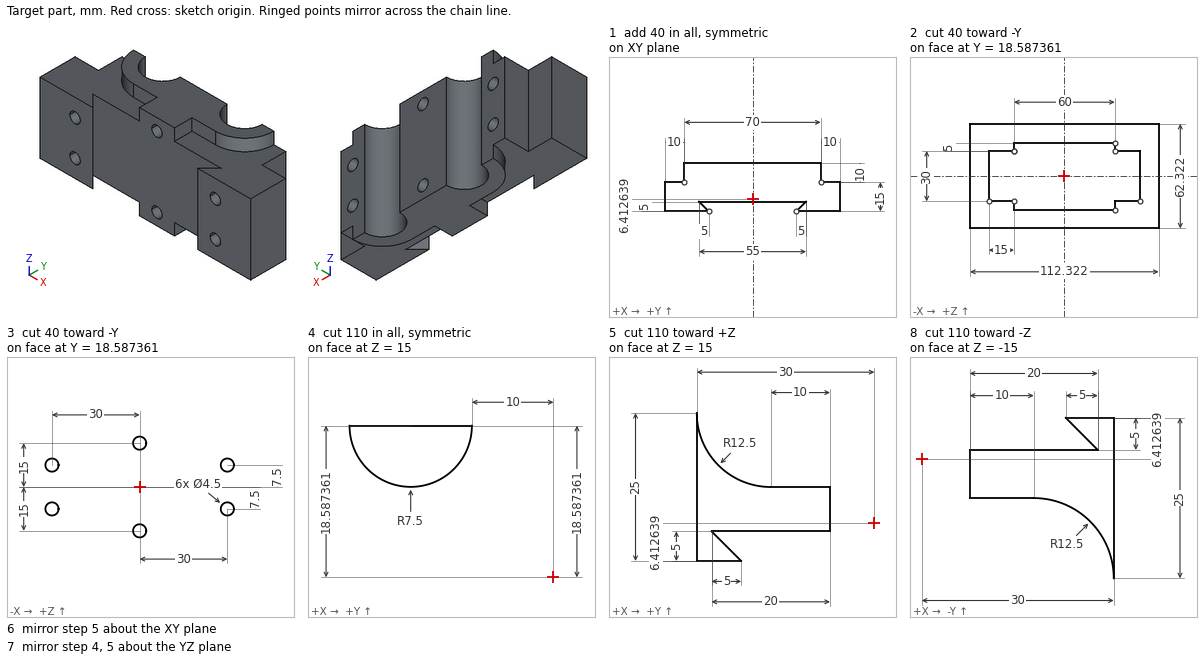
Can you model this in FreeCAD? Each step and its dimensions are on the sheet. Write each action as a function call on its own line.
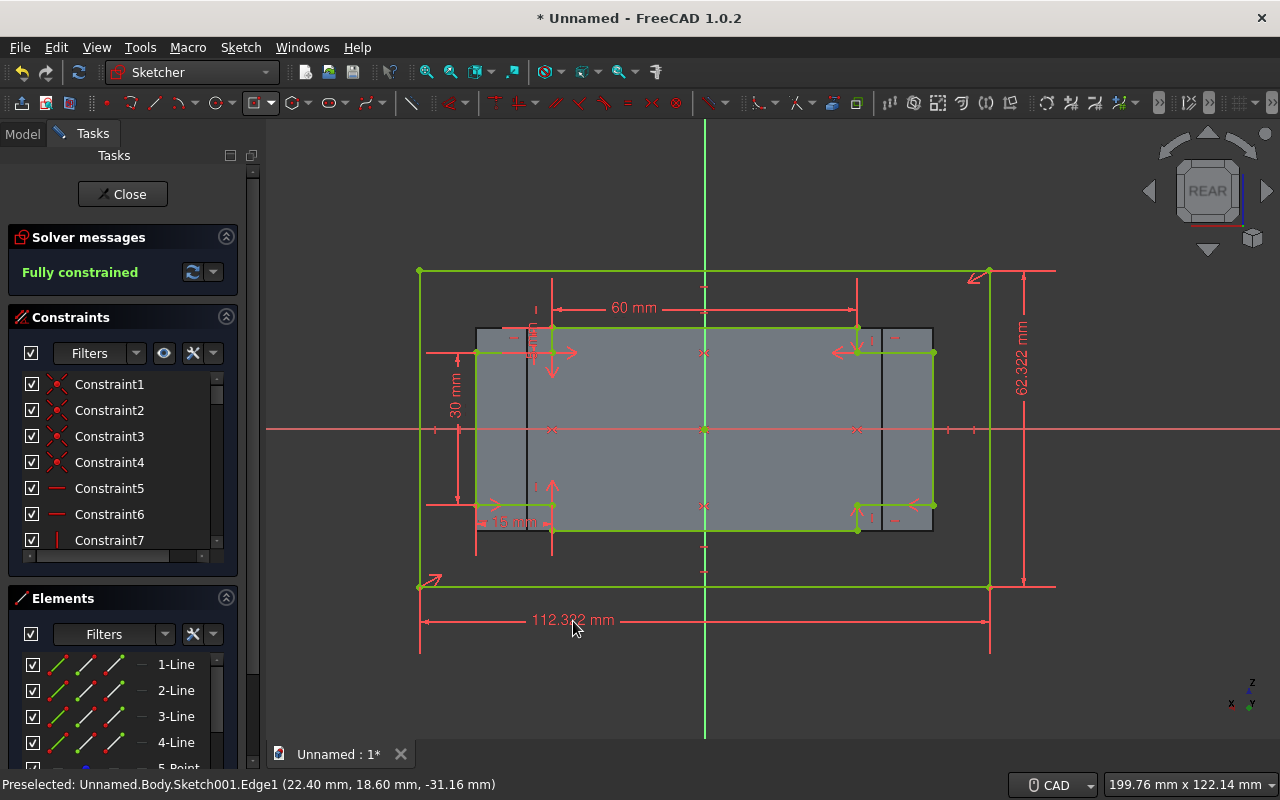
click(123, 194)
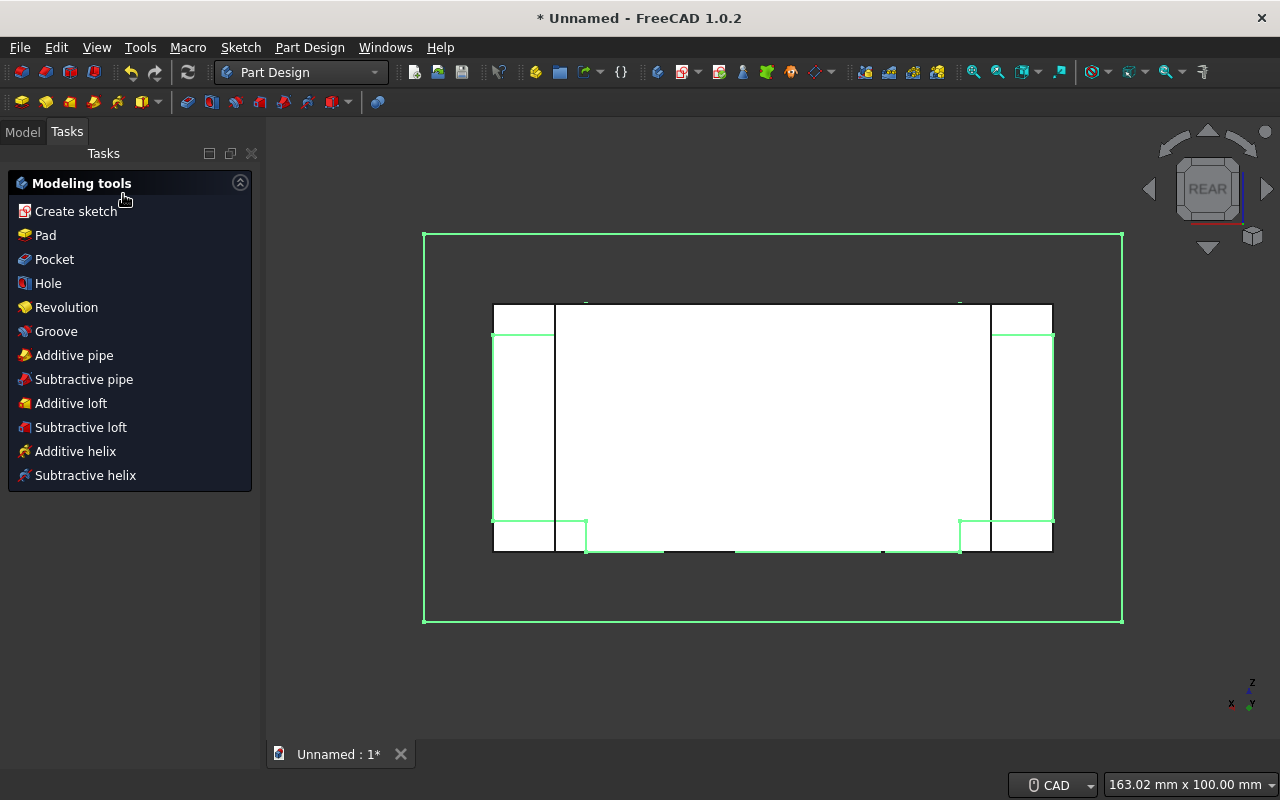
click(188, 102)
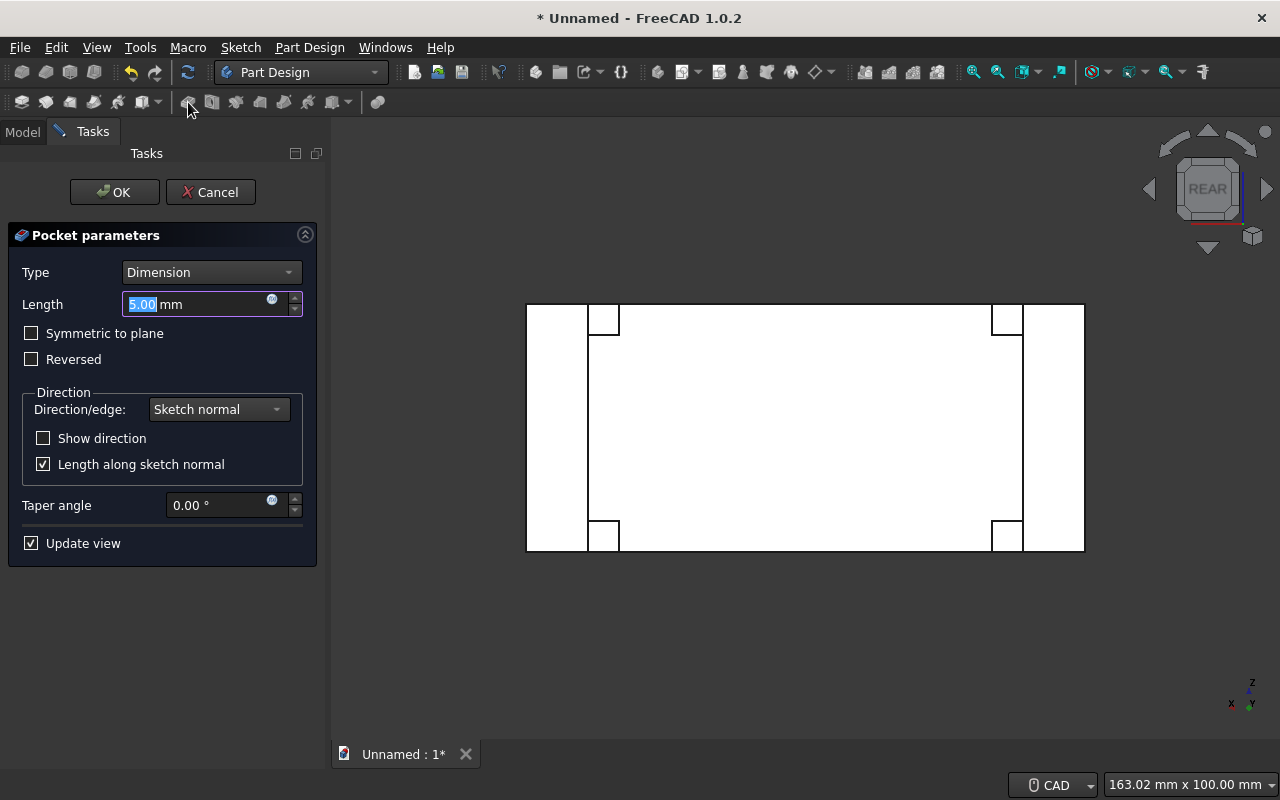
text(40)
key(Tab)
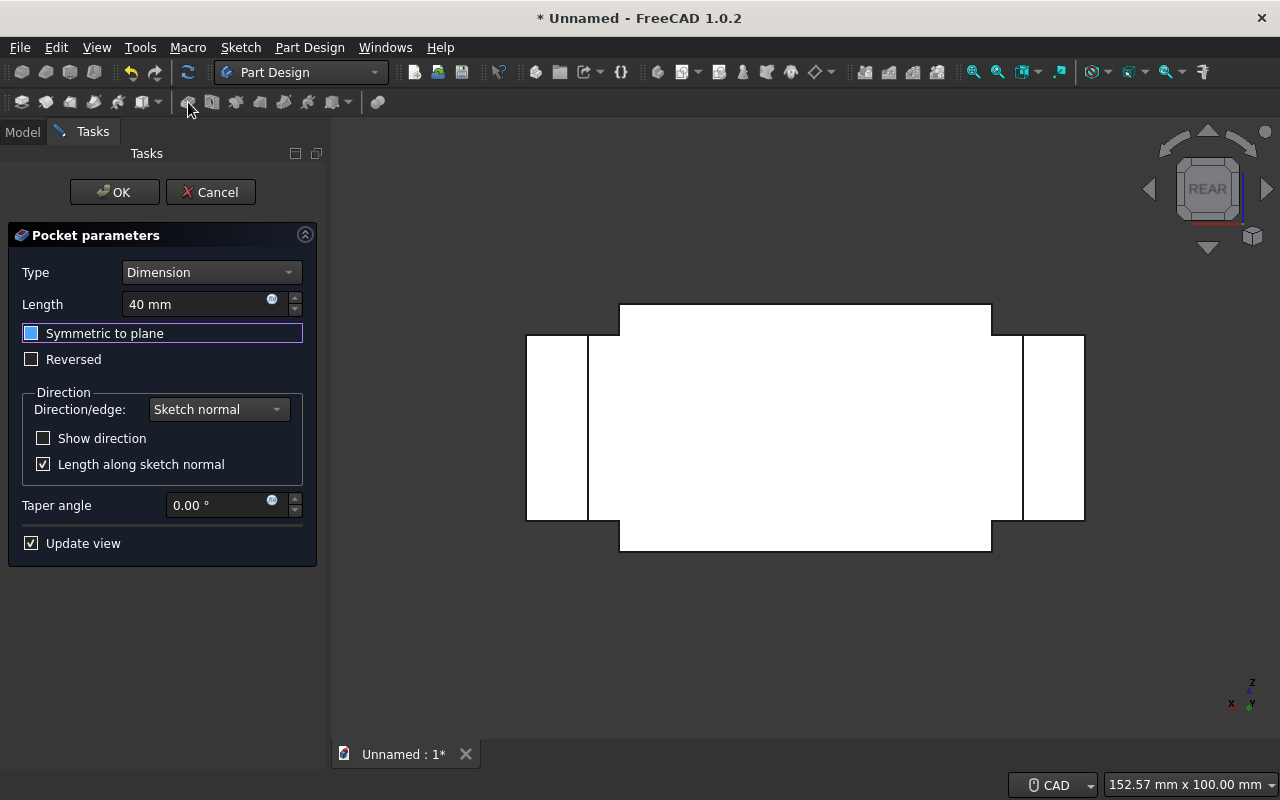
click(115, 192)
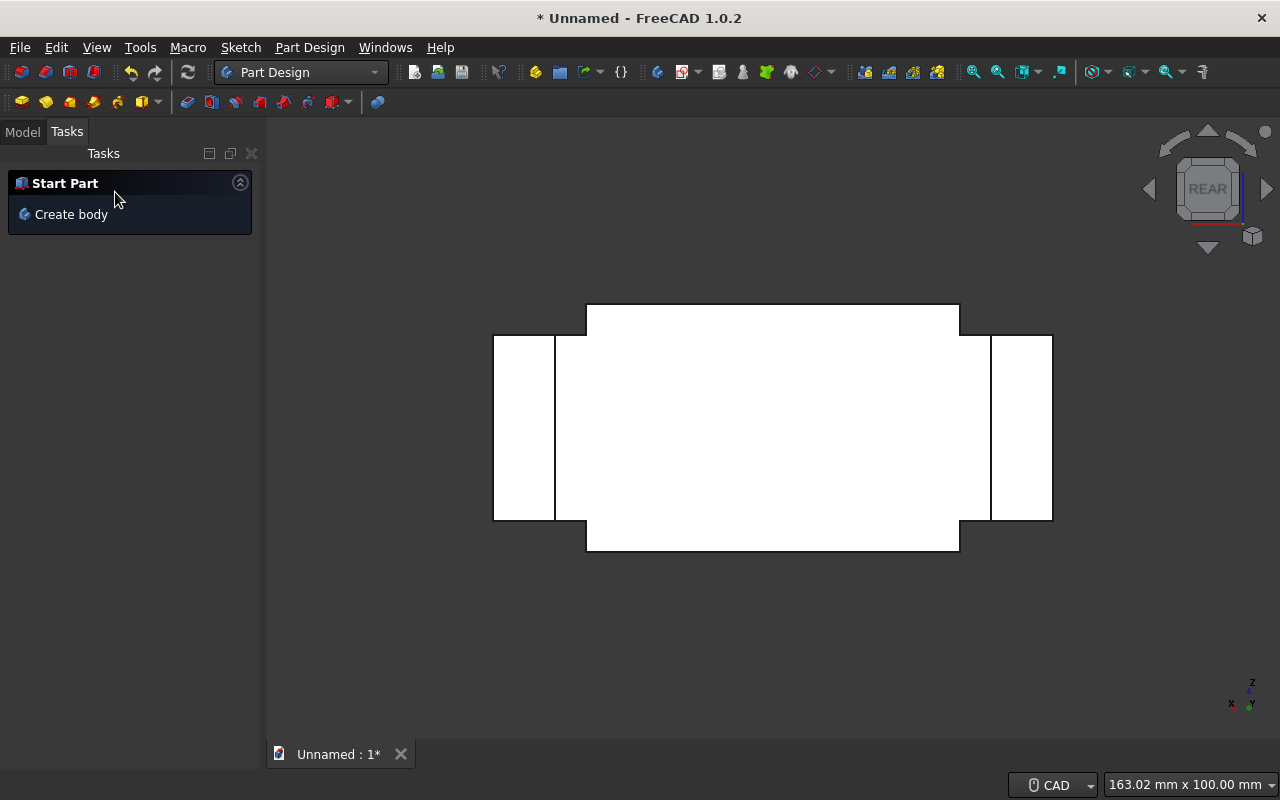
click(711, 427)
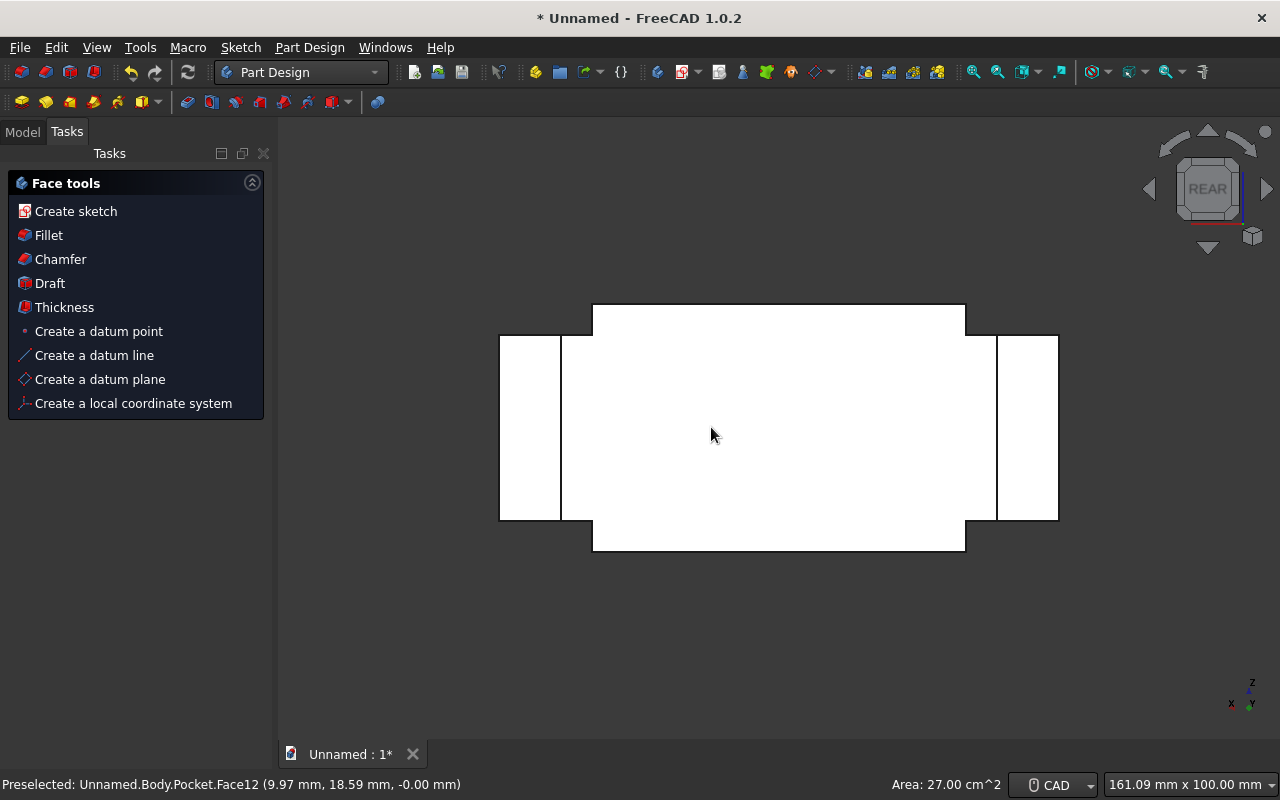
click(682, 72)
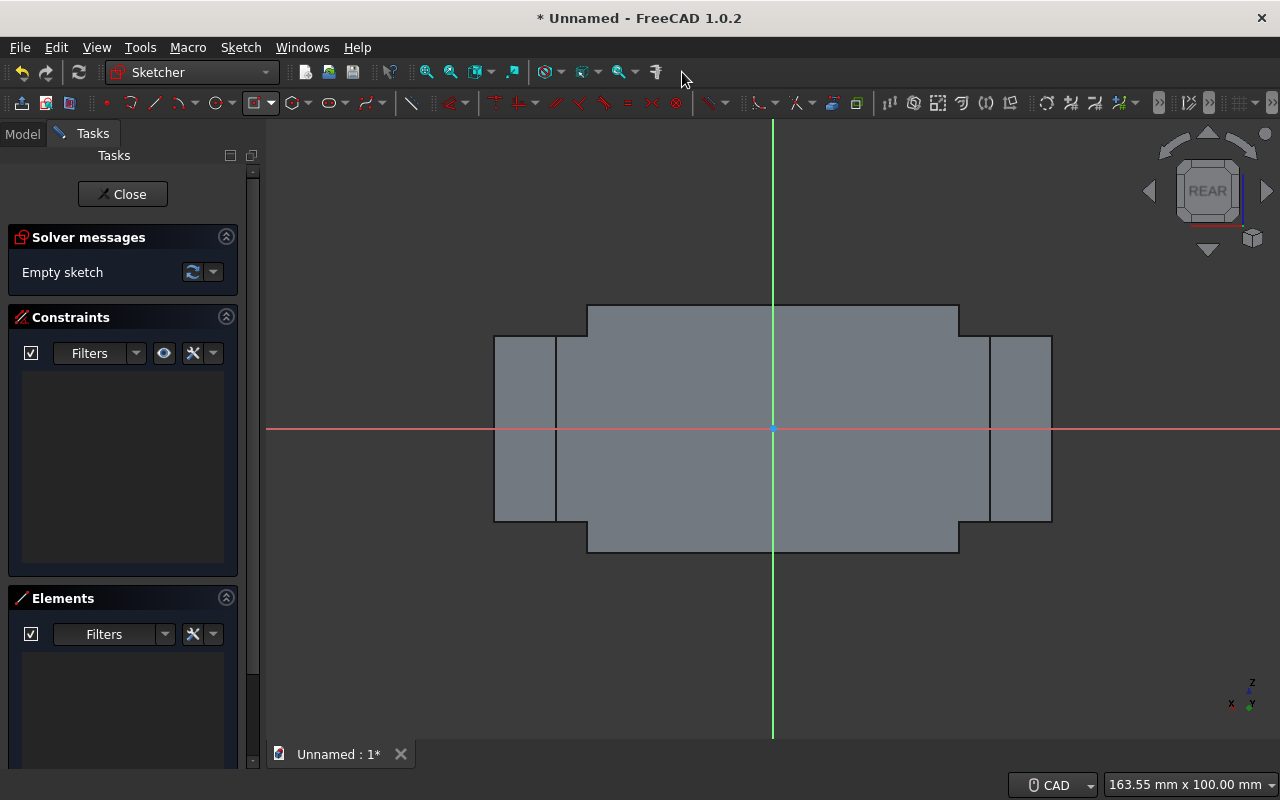
scroll(912, 429, up, 2)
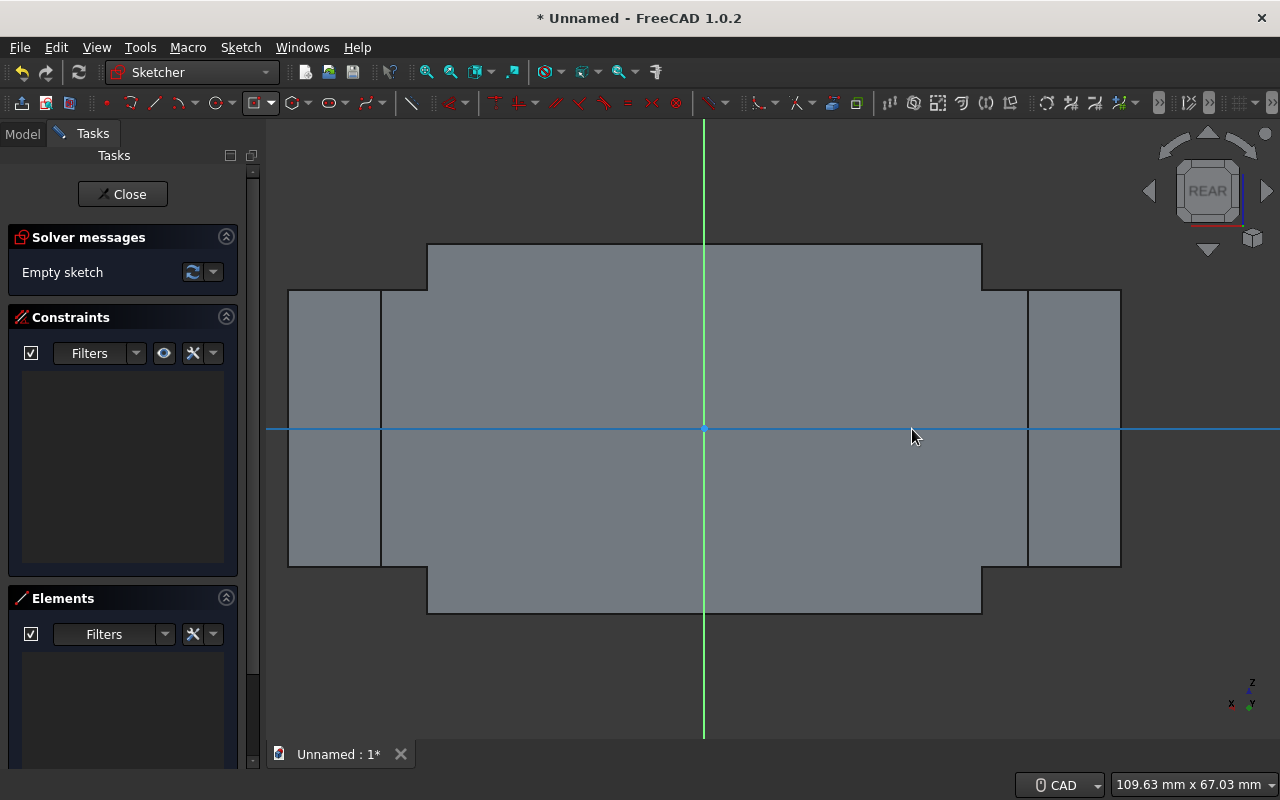
key(g)
key(c)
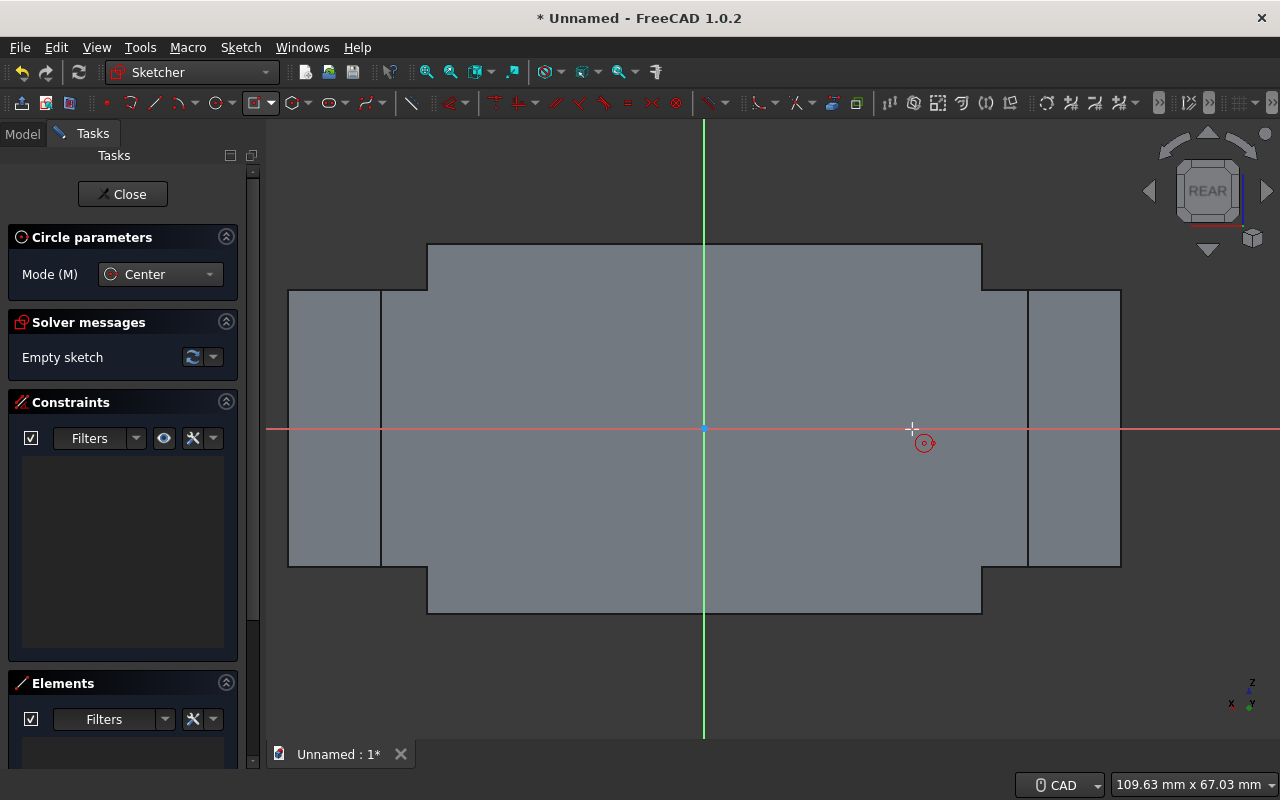
click(982, 498)
click(997, 483)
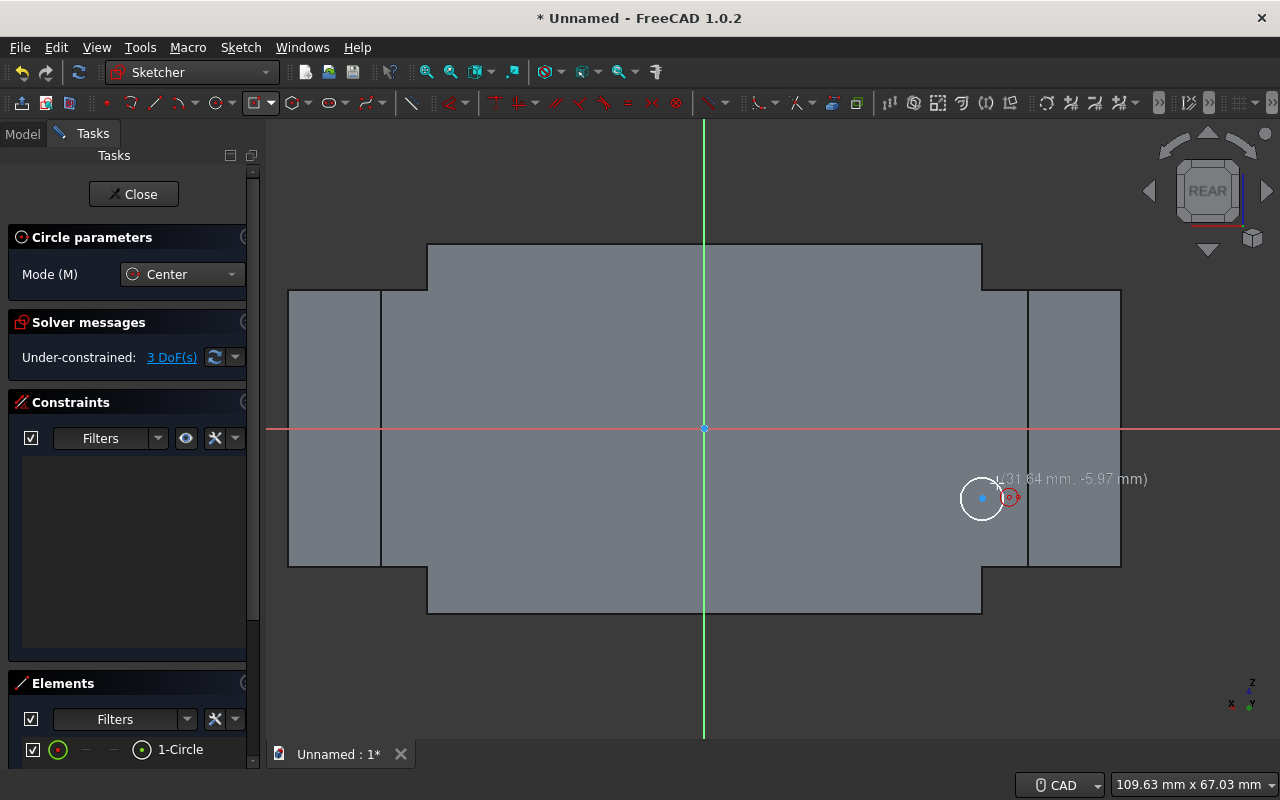
click(982, 359)
click(997, 345)